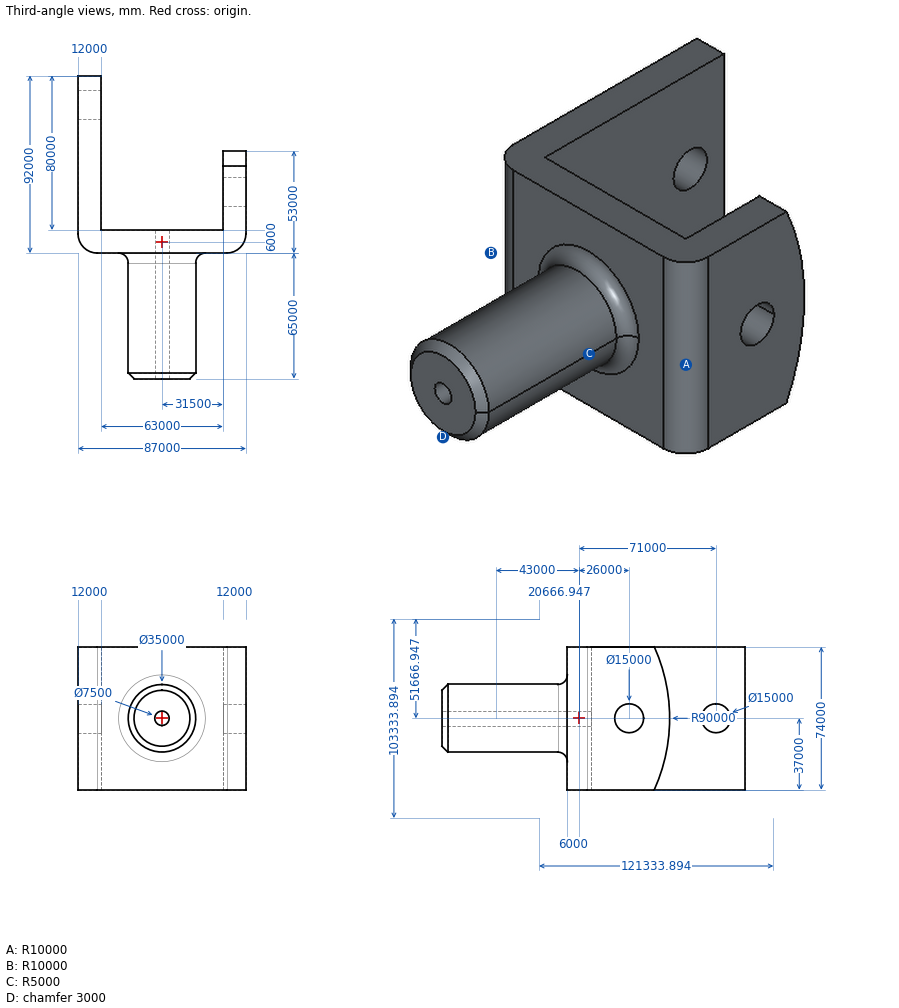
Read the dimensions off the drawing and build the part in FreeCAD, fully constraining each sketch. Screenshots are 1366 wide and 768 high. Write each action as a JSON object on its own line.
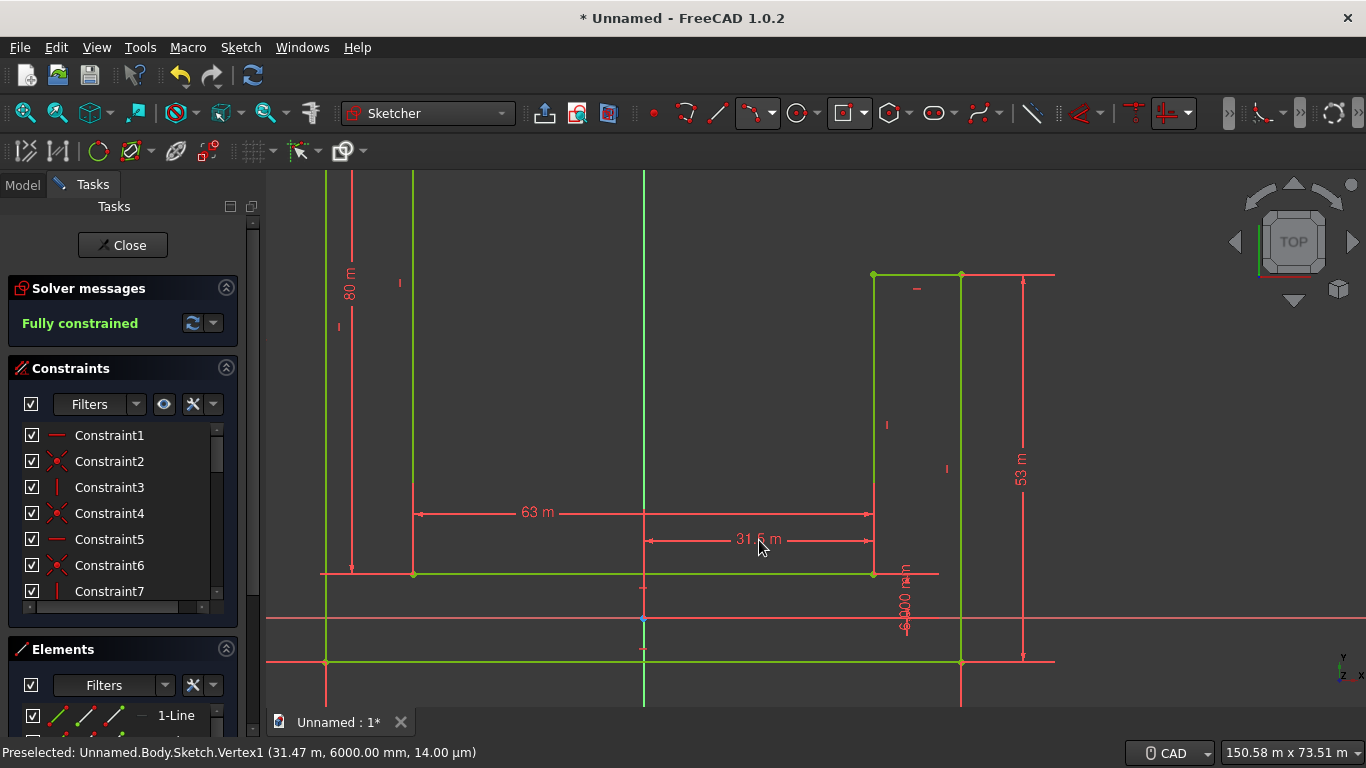
{"action": "left_click", "coordinate": [123, 245]}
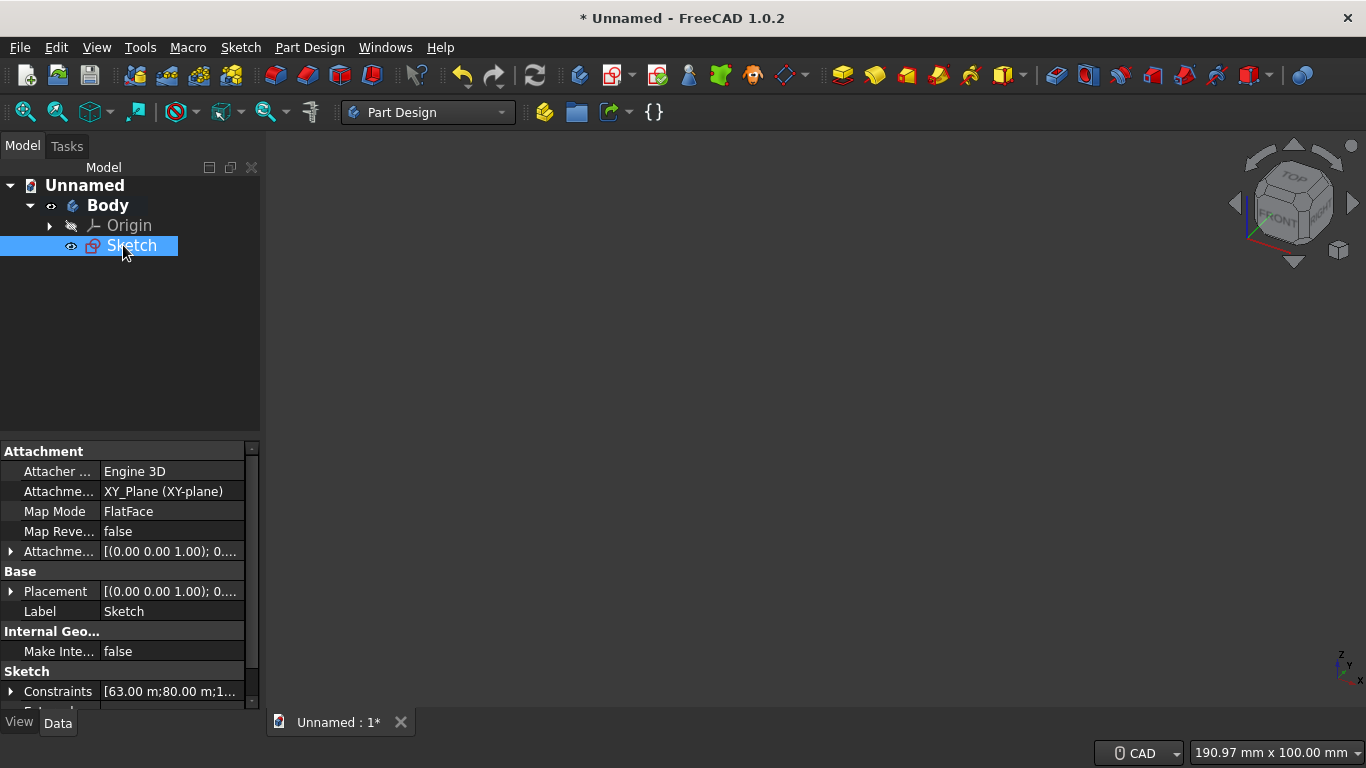
{"action": "left_click", "coordinate": [844, 76]}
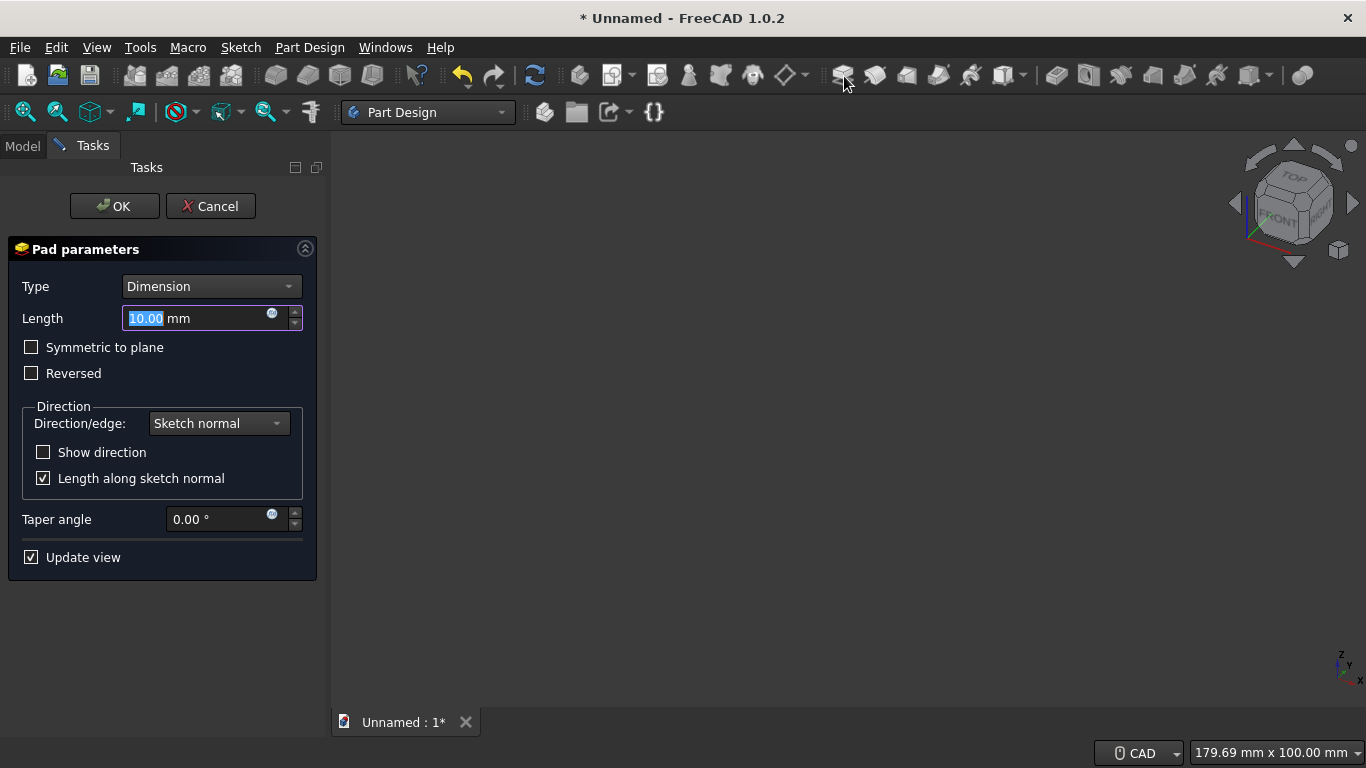
{"action": "type", "text": "74000"}
{"action": "key", "text": "Tab"}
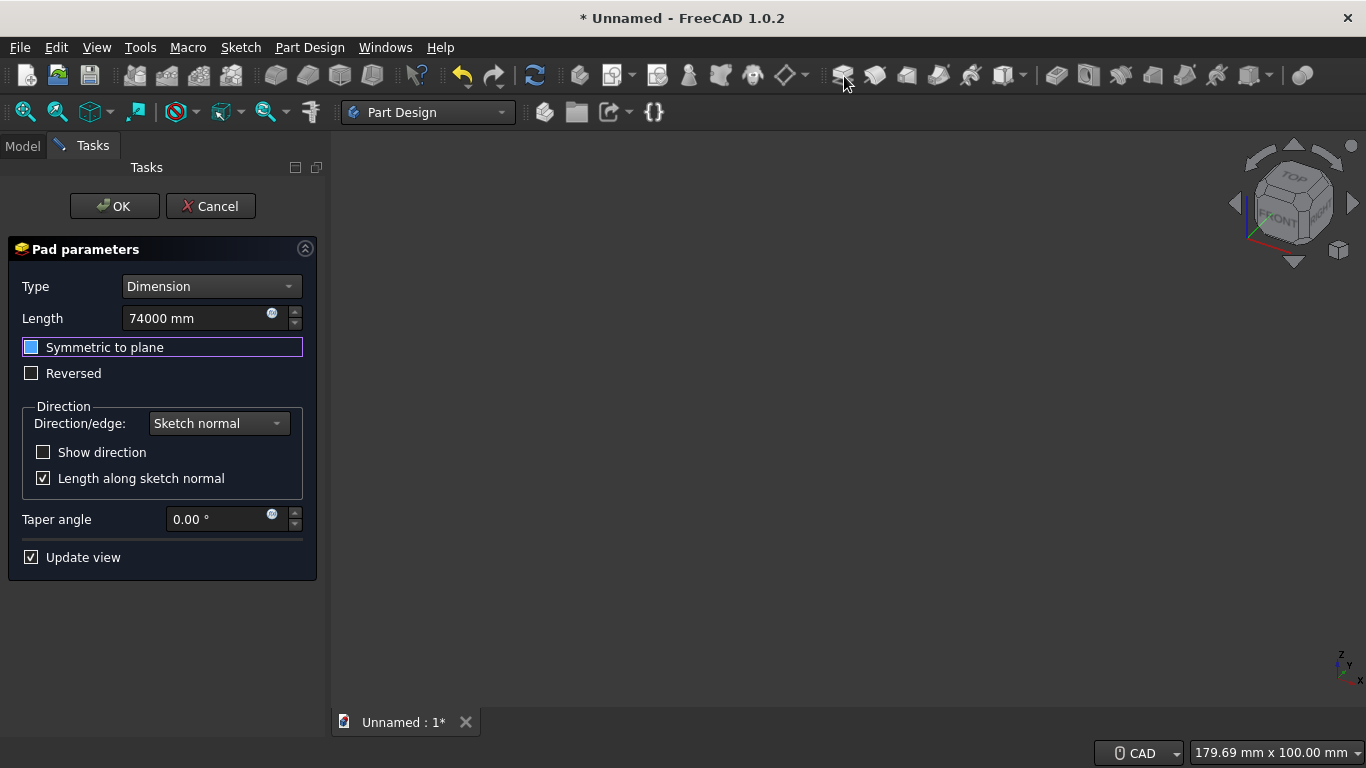
{"action": "left_click", "coordinate": [30, 347]}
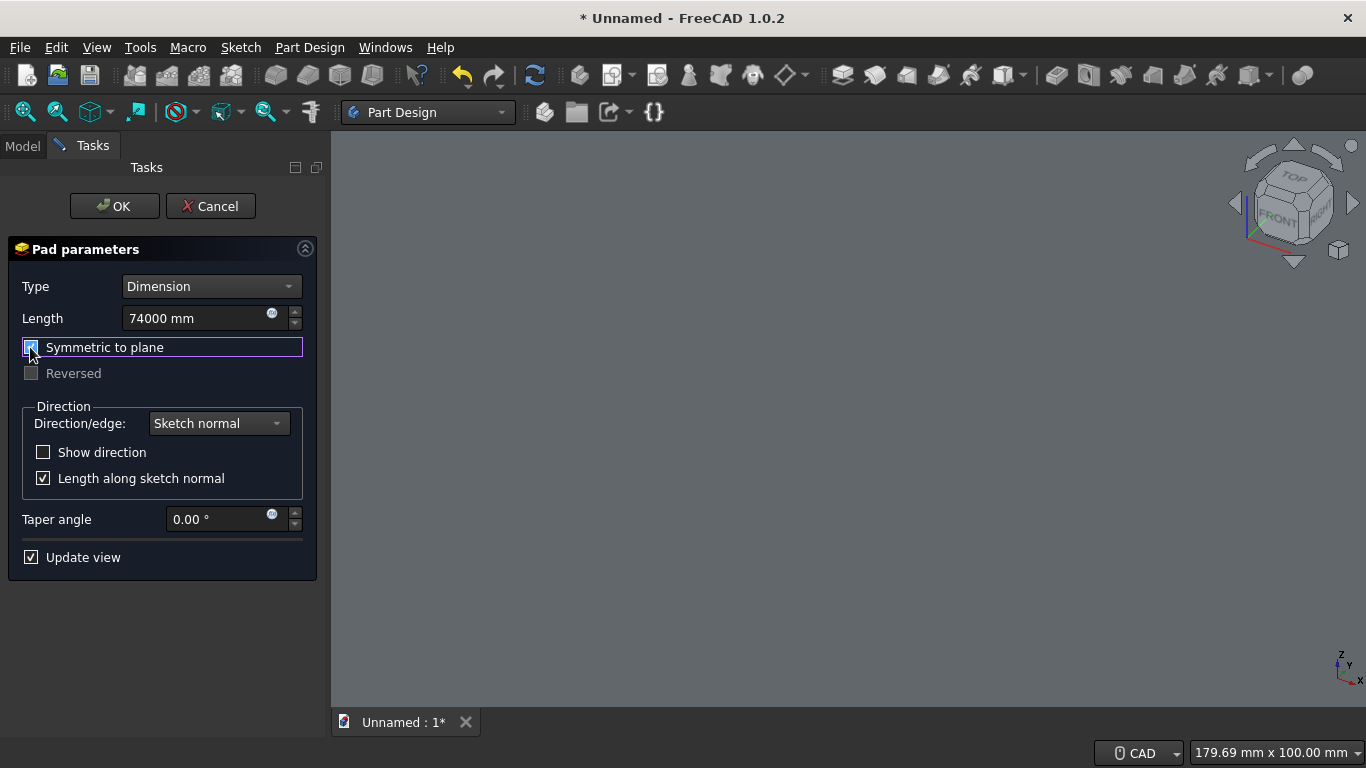
{"action": "left_click", "coordinate": [115, 206]}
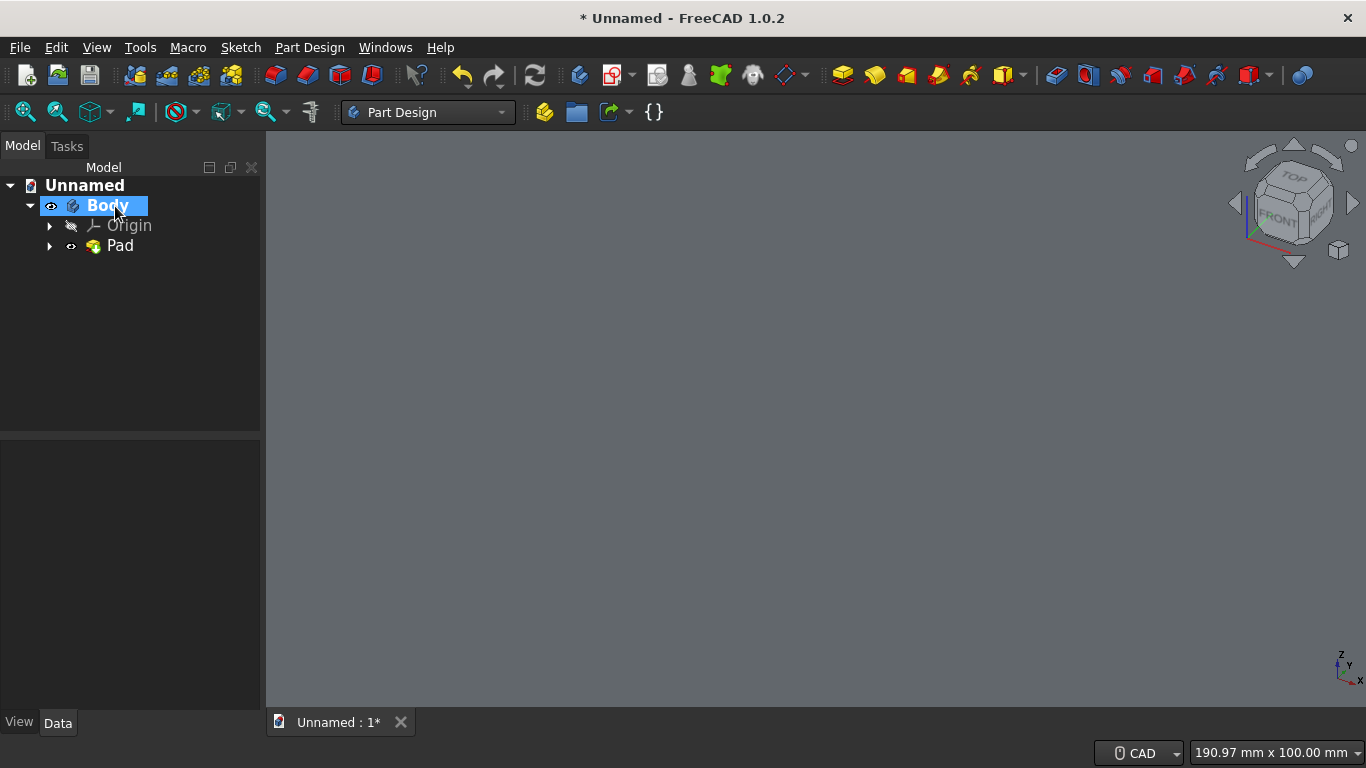
{"action": "left_click", "coordinate": [26, 112]}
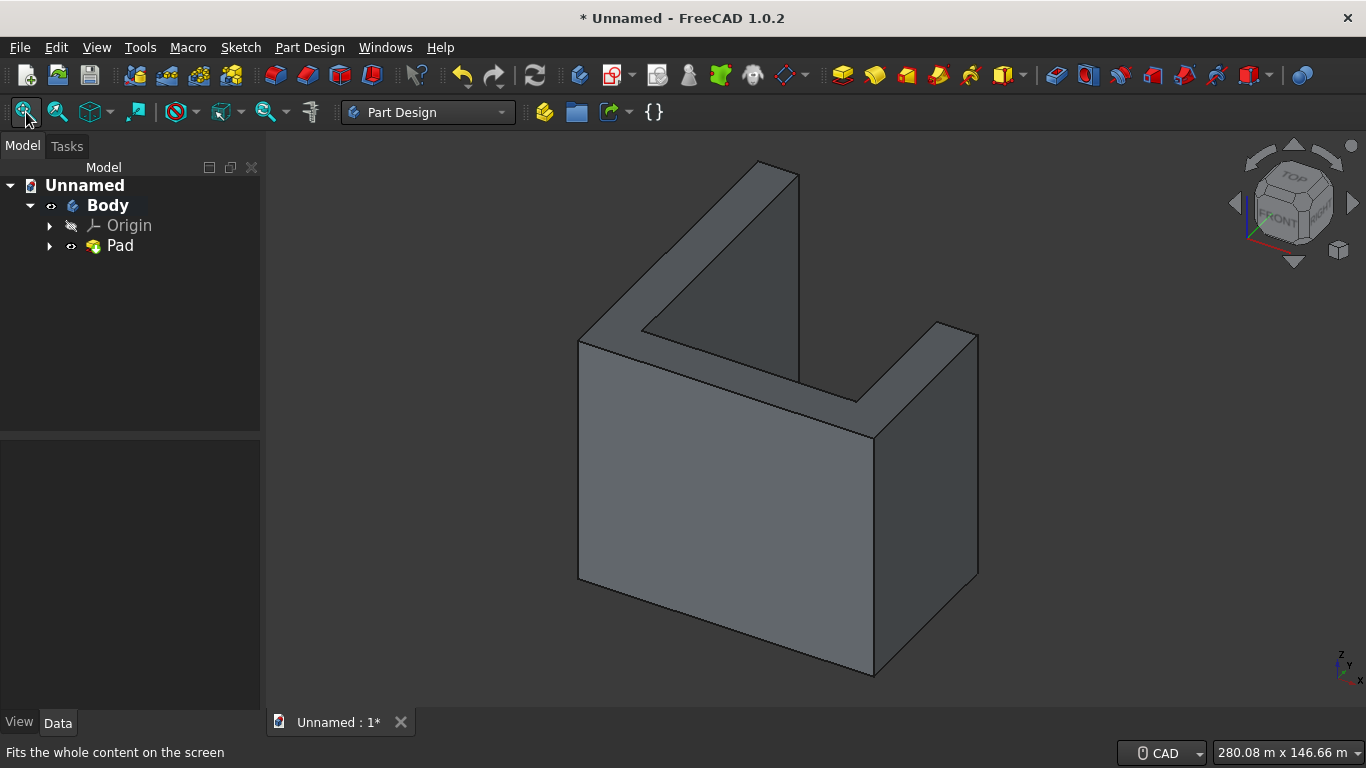
{"action": "left_click", "coordinate": [874, 557]}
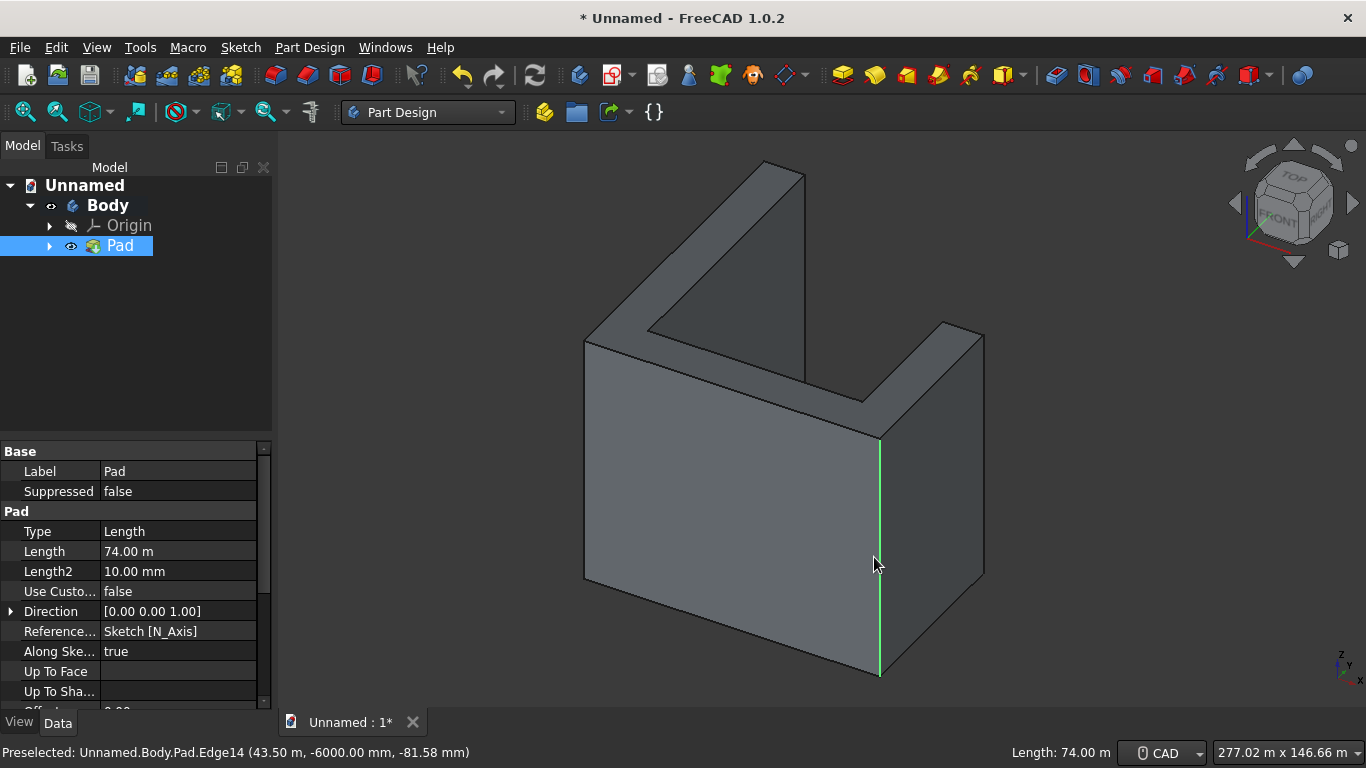
{"action": "left_click", "coordinate": [276, 76]}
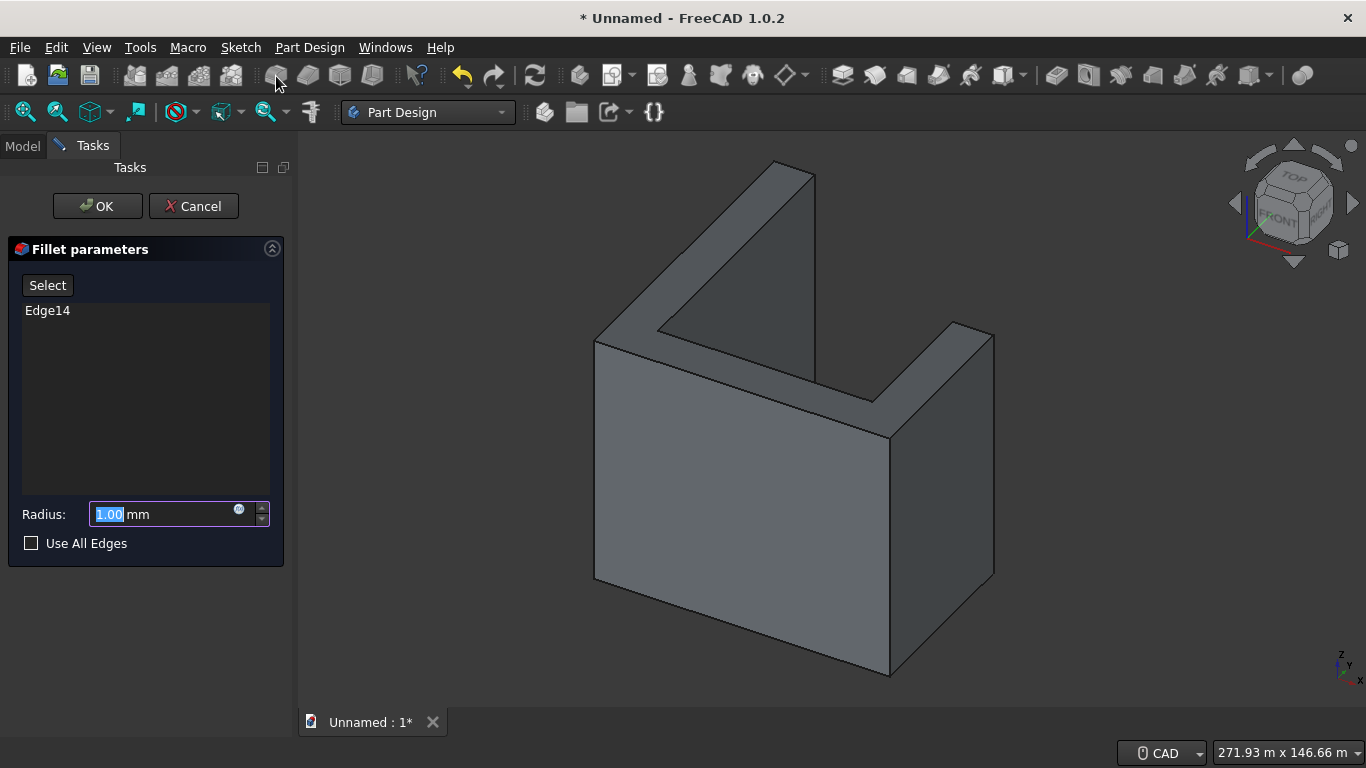
{"action": "type", "text": "10000"}
{"action": "key", "text": "Tab"}